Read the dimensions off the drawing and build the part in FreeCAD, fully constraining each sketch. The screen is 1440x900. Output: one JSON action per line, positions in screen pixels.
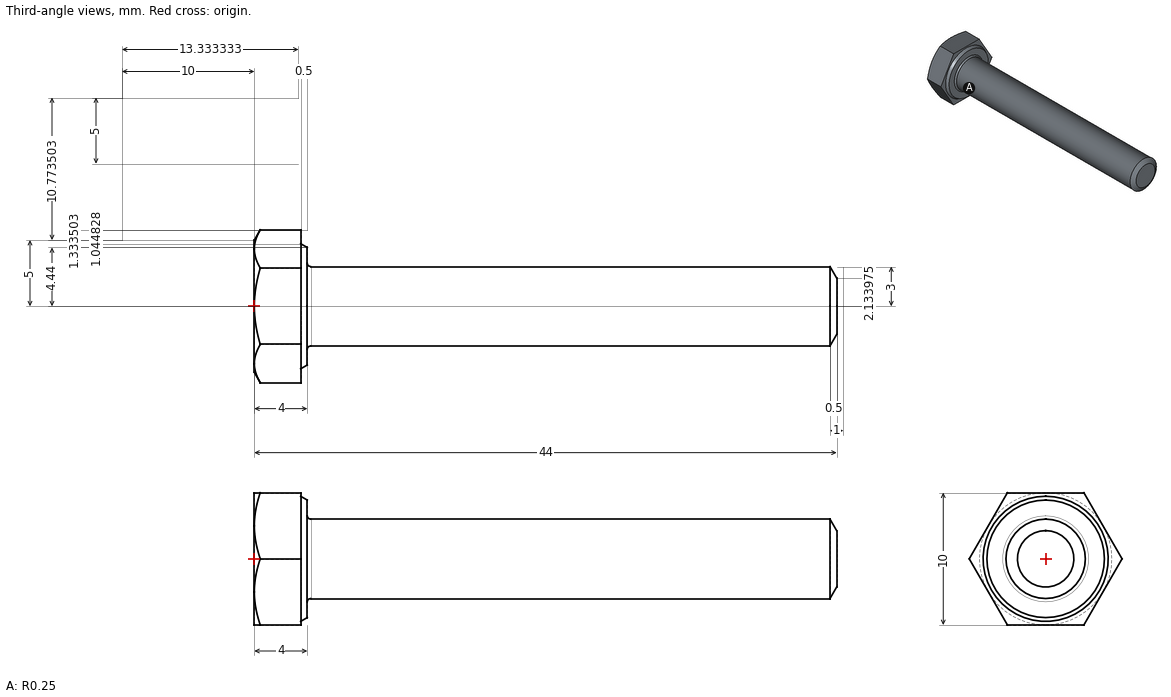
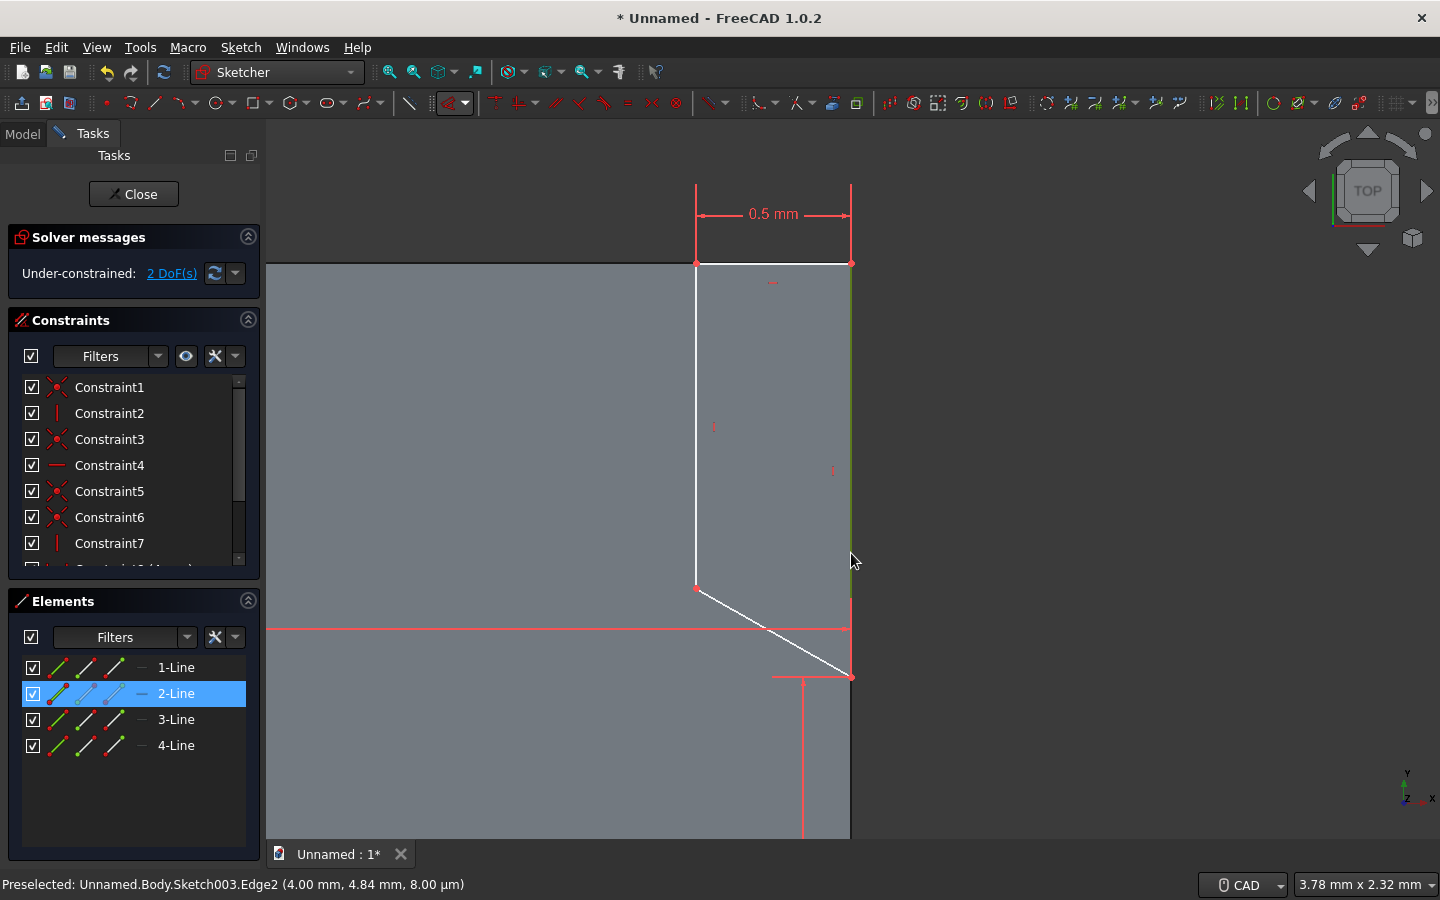
{"action": "key", "text": "i"}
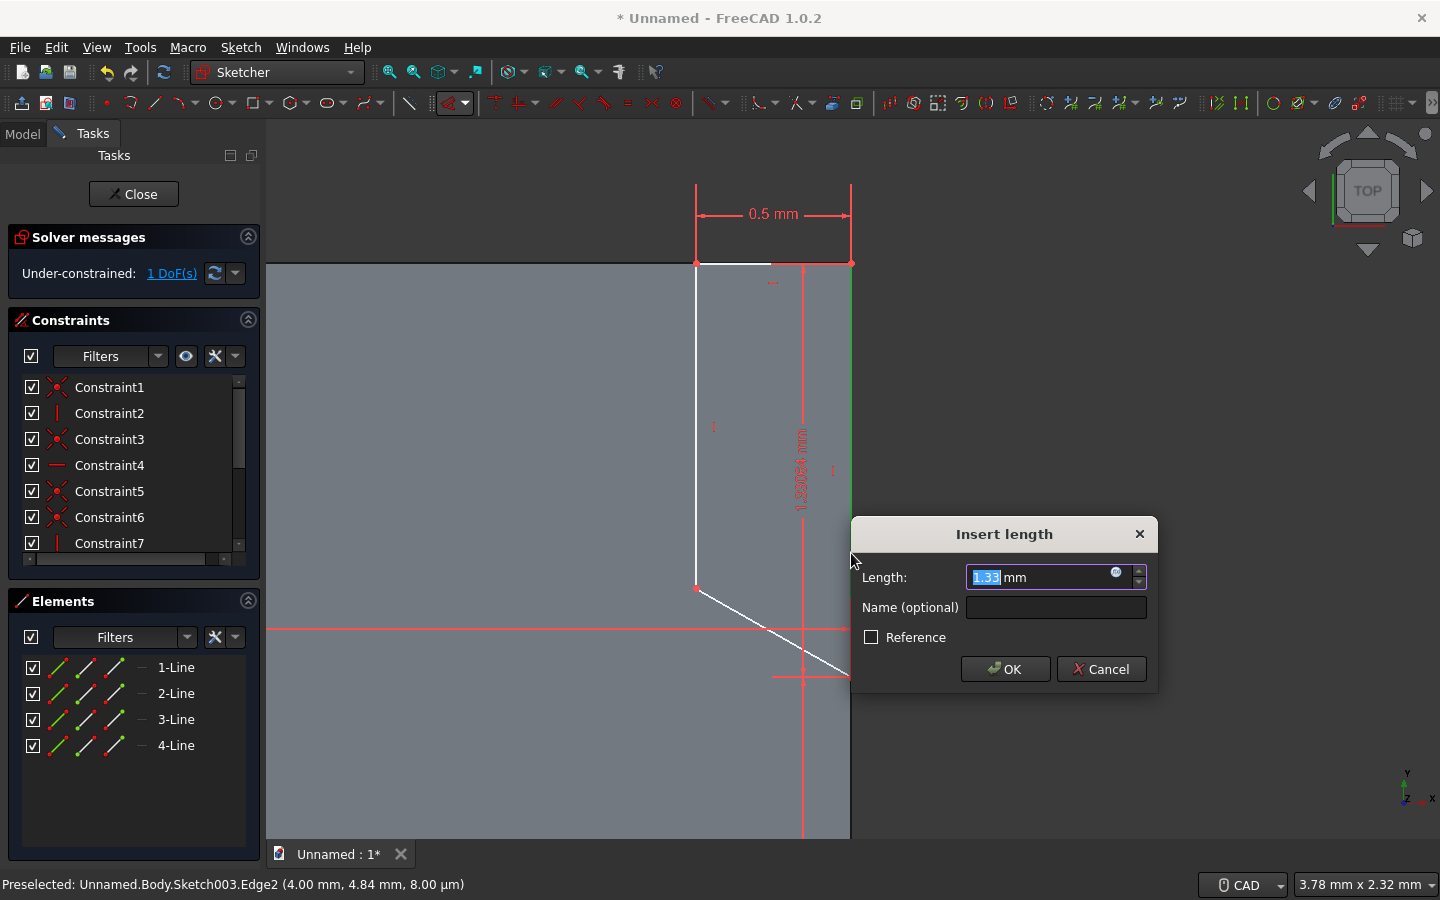
{"action": "type", "text": "1.333503"}
{"action": "key", "text": "Return"}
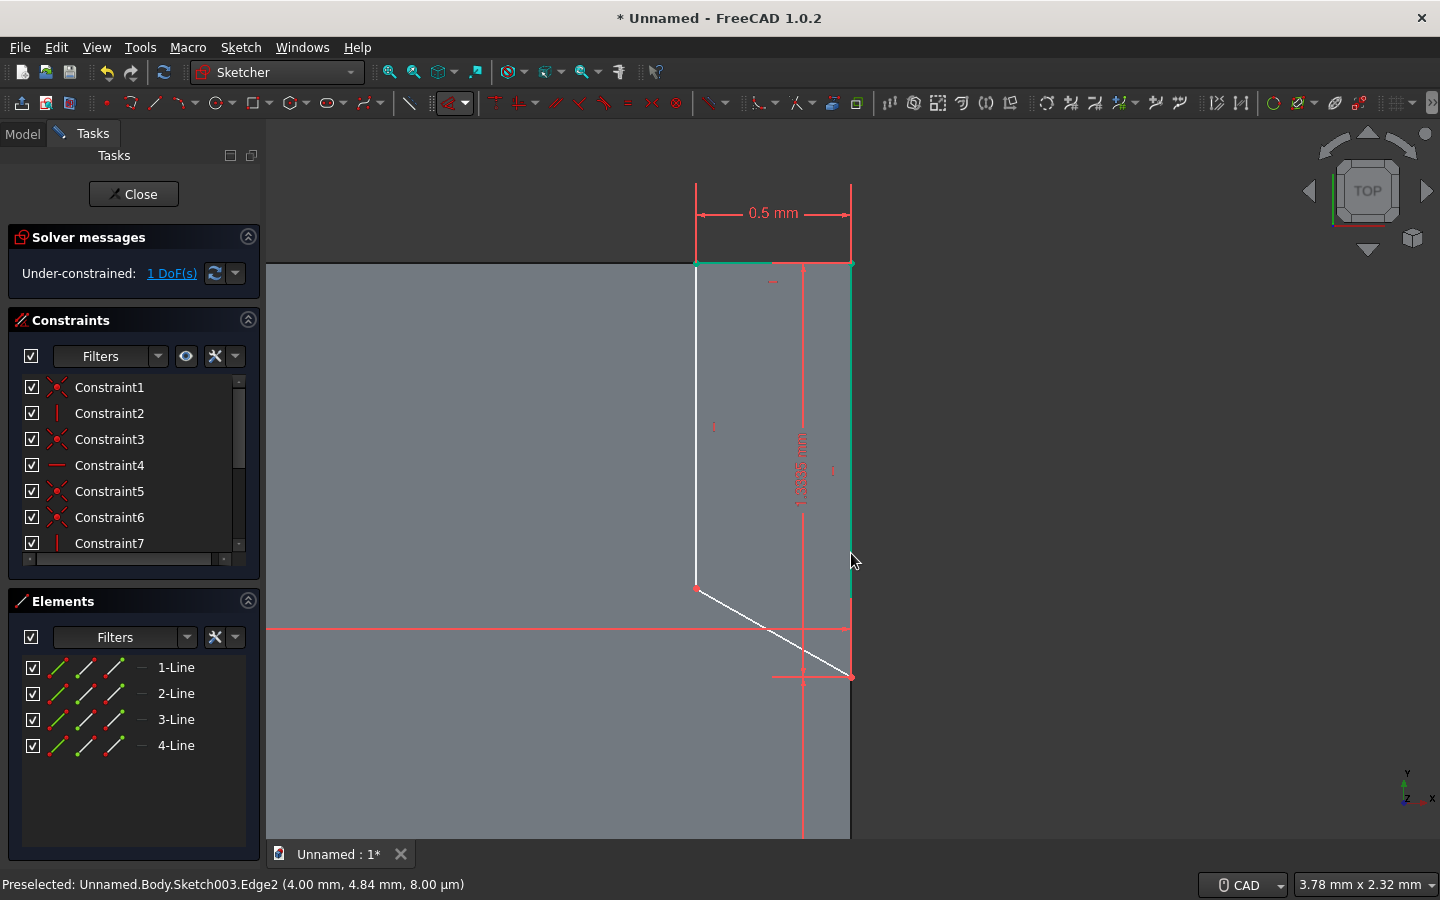
{"action": "left_click", "coordinate": [696, 361]}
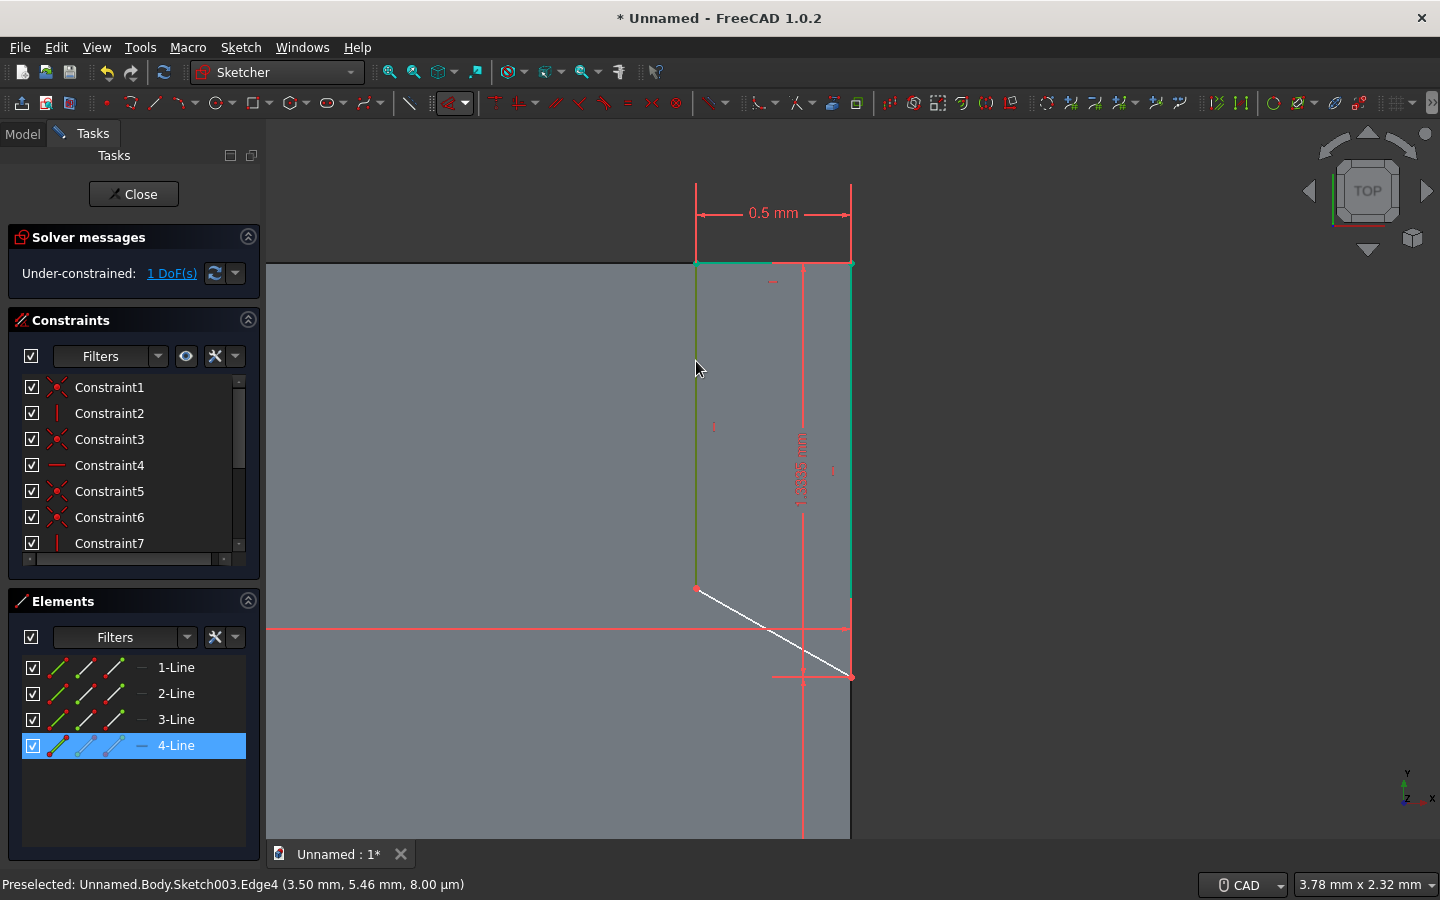
{"action": "key", "text": "i"}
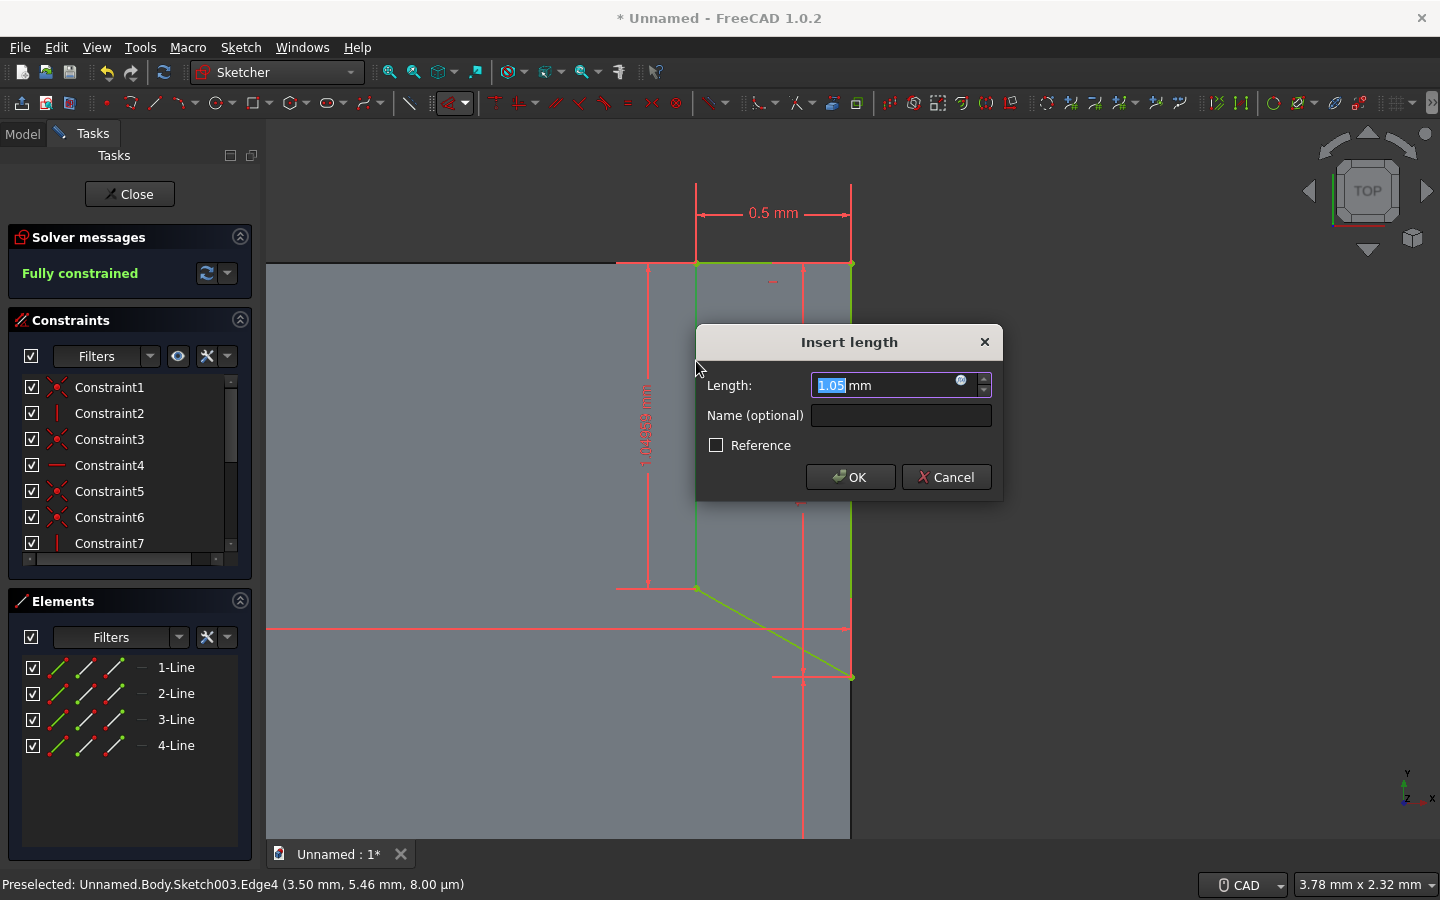
{"action": "type", "text": "1.044828"}
{"action": "key", "text": "Return"}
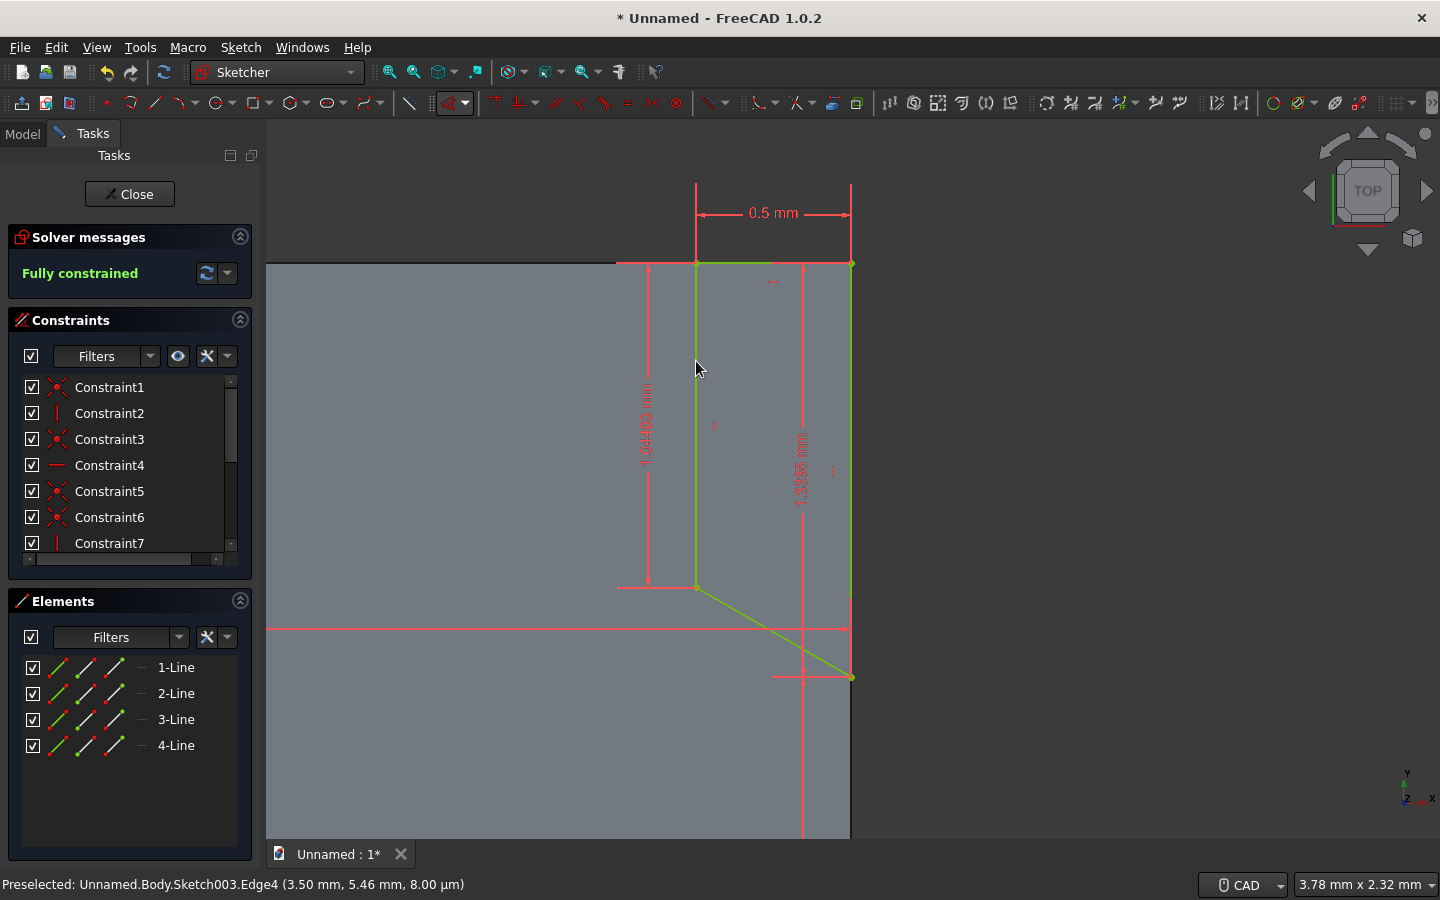
{"action": "left_click", "coordinate": [130, 194]}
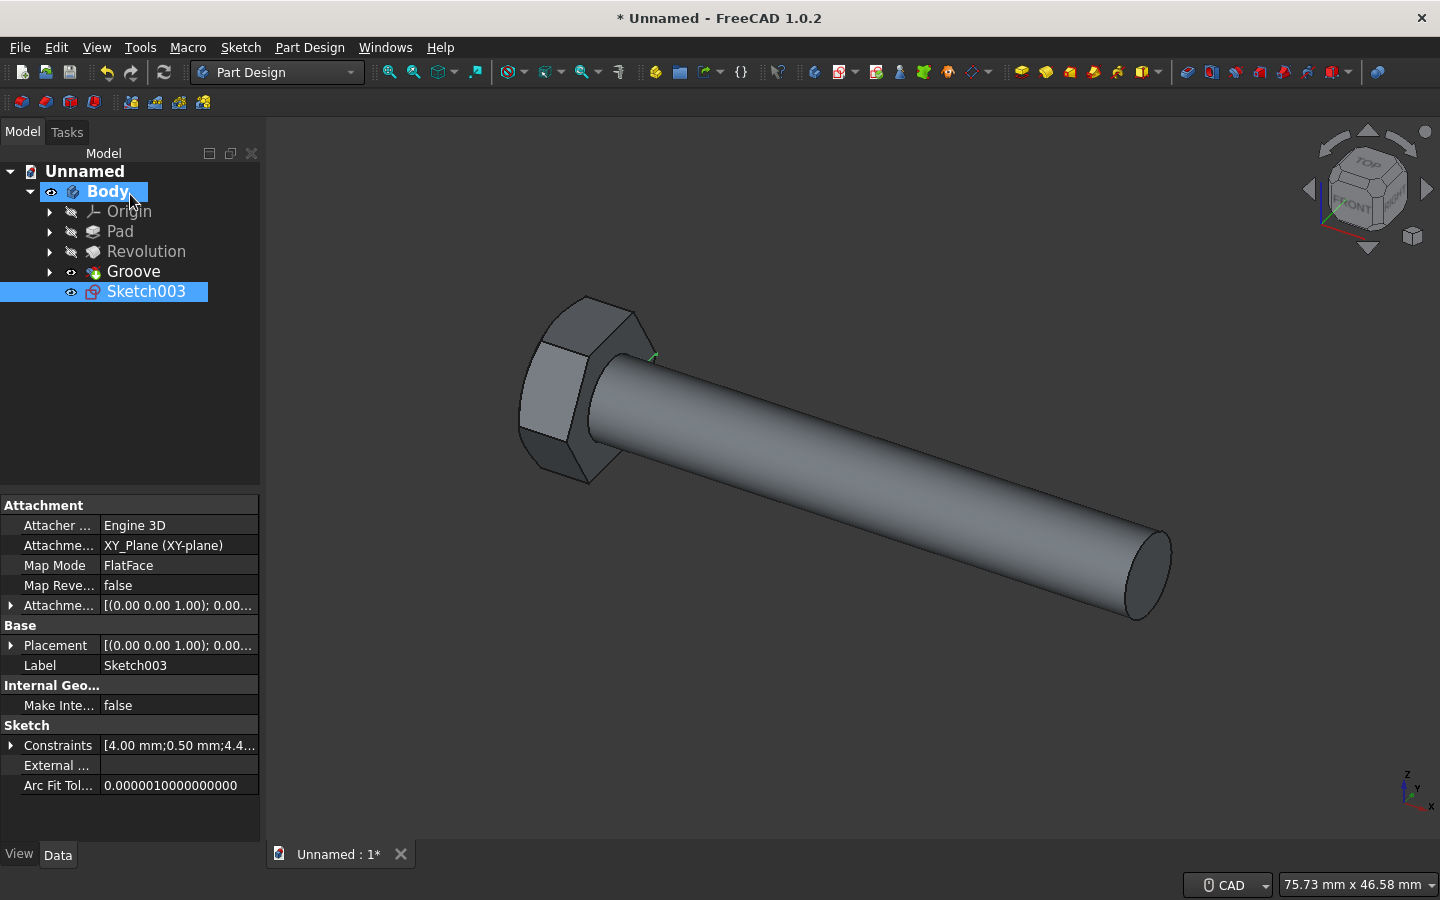
{"action": "left_click", "coordinate": [1236, 72]}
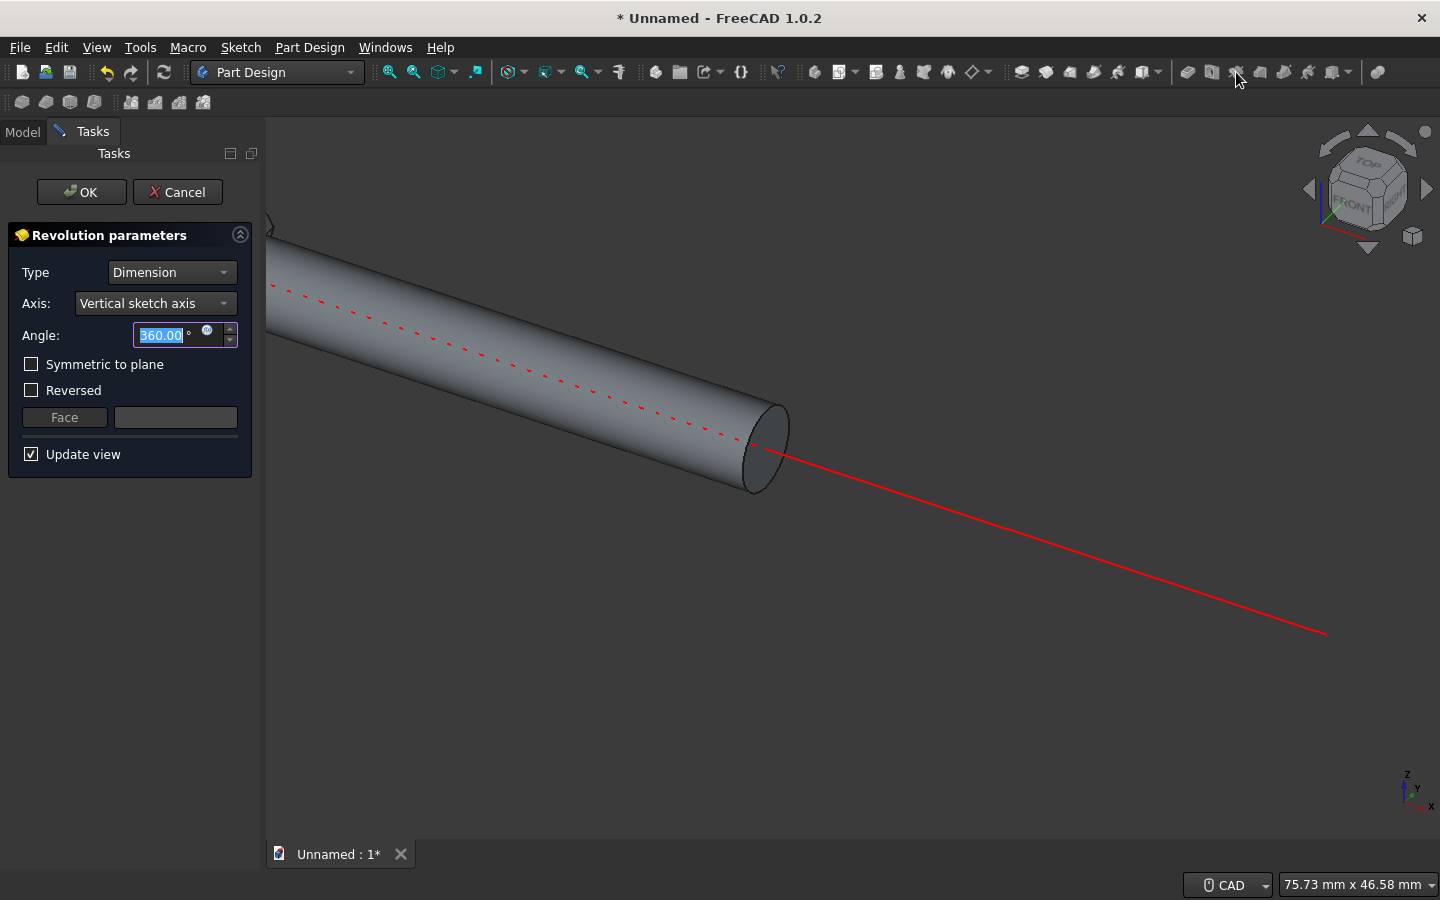
{"action": "left_click", "coordinate": [156, 304]}